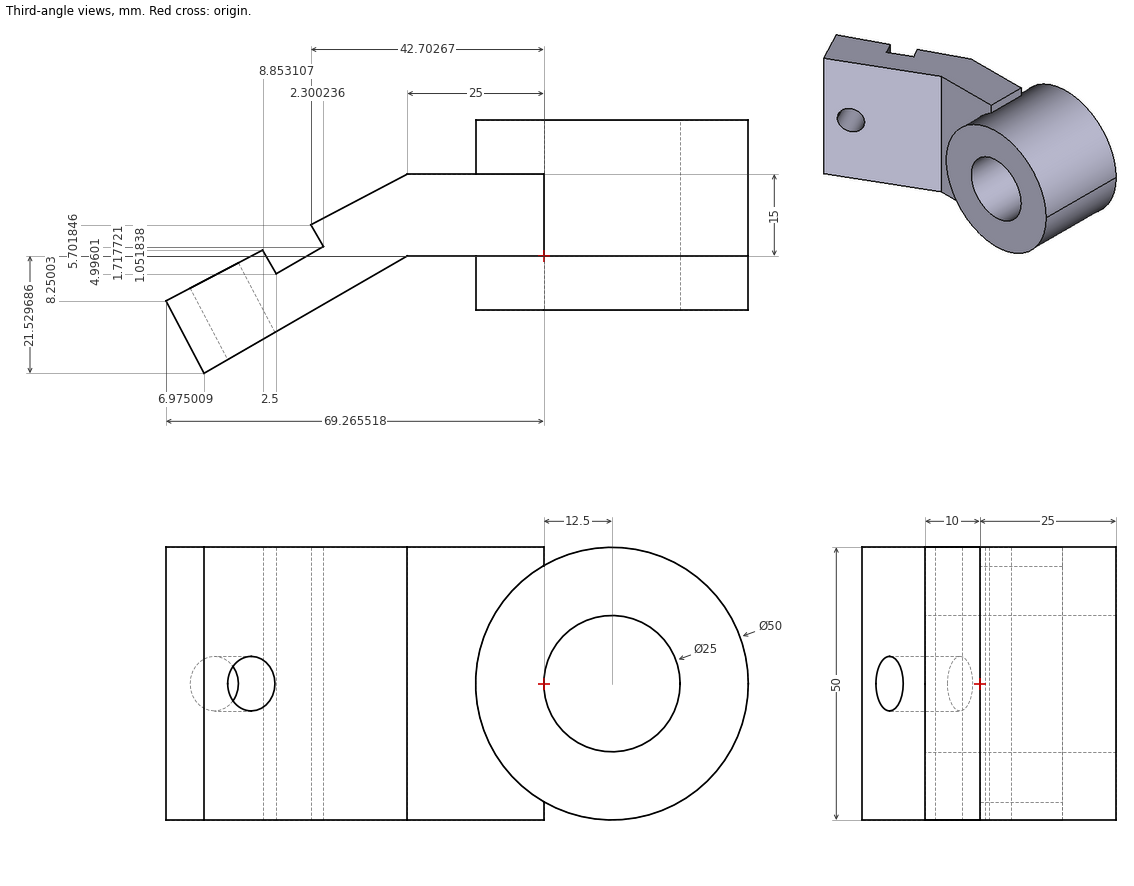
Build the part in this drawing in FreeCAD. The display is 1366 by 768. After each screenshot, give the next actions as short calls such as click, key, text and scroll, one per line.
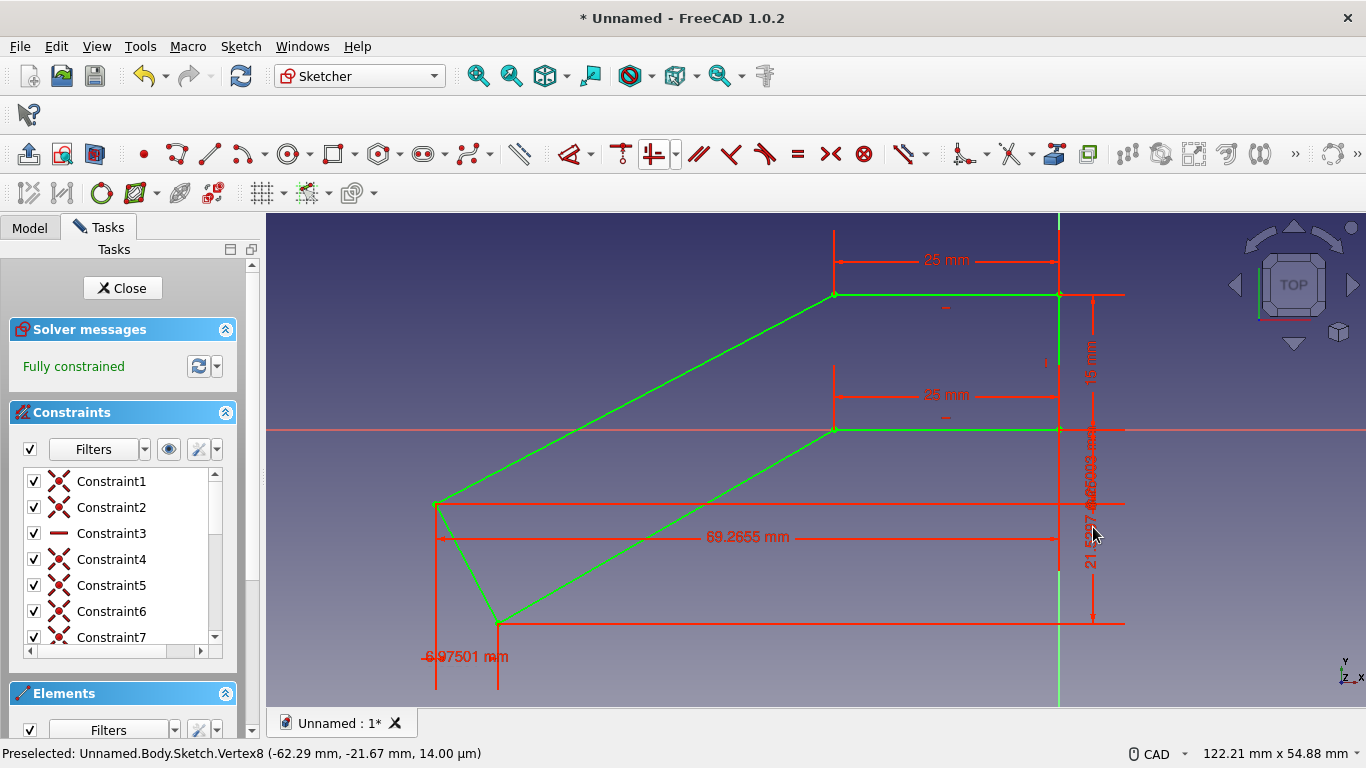
click(123, 288)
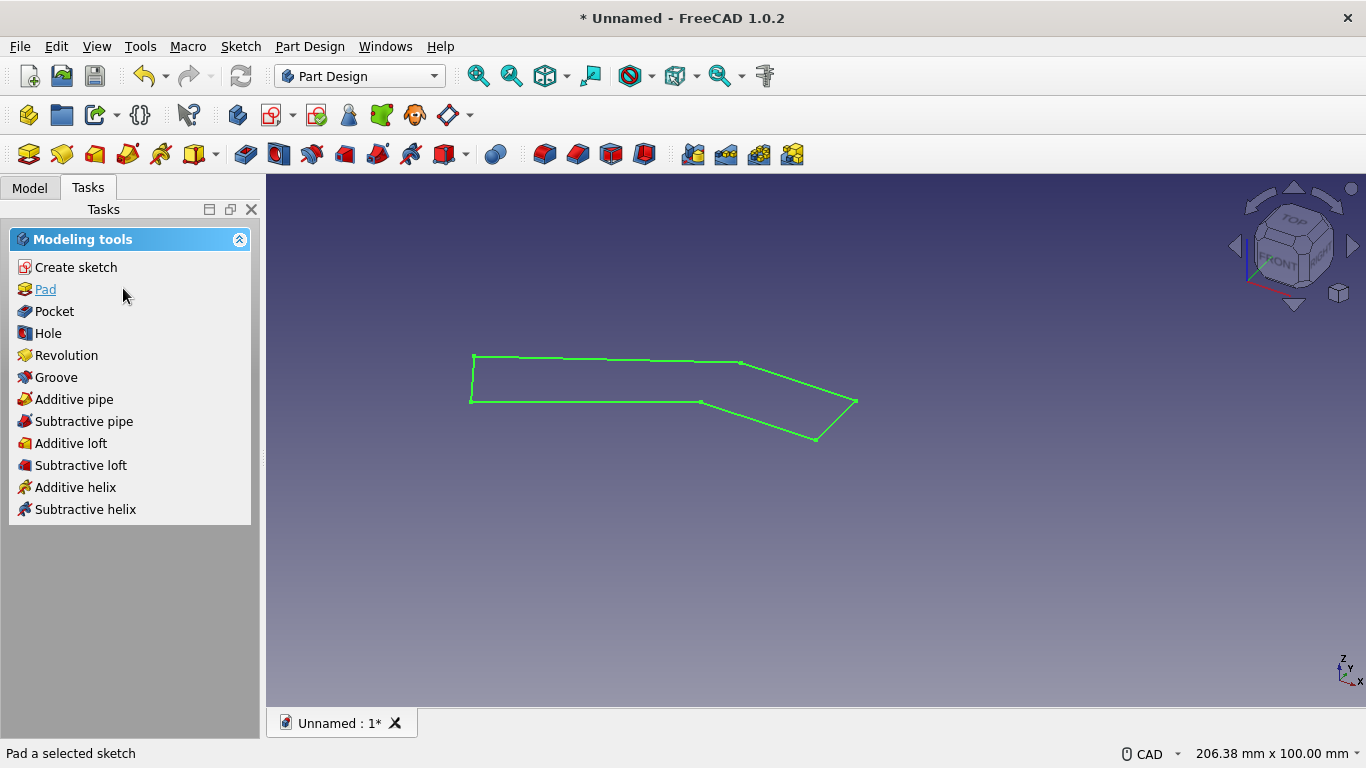
click(29, 154)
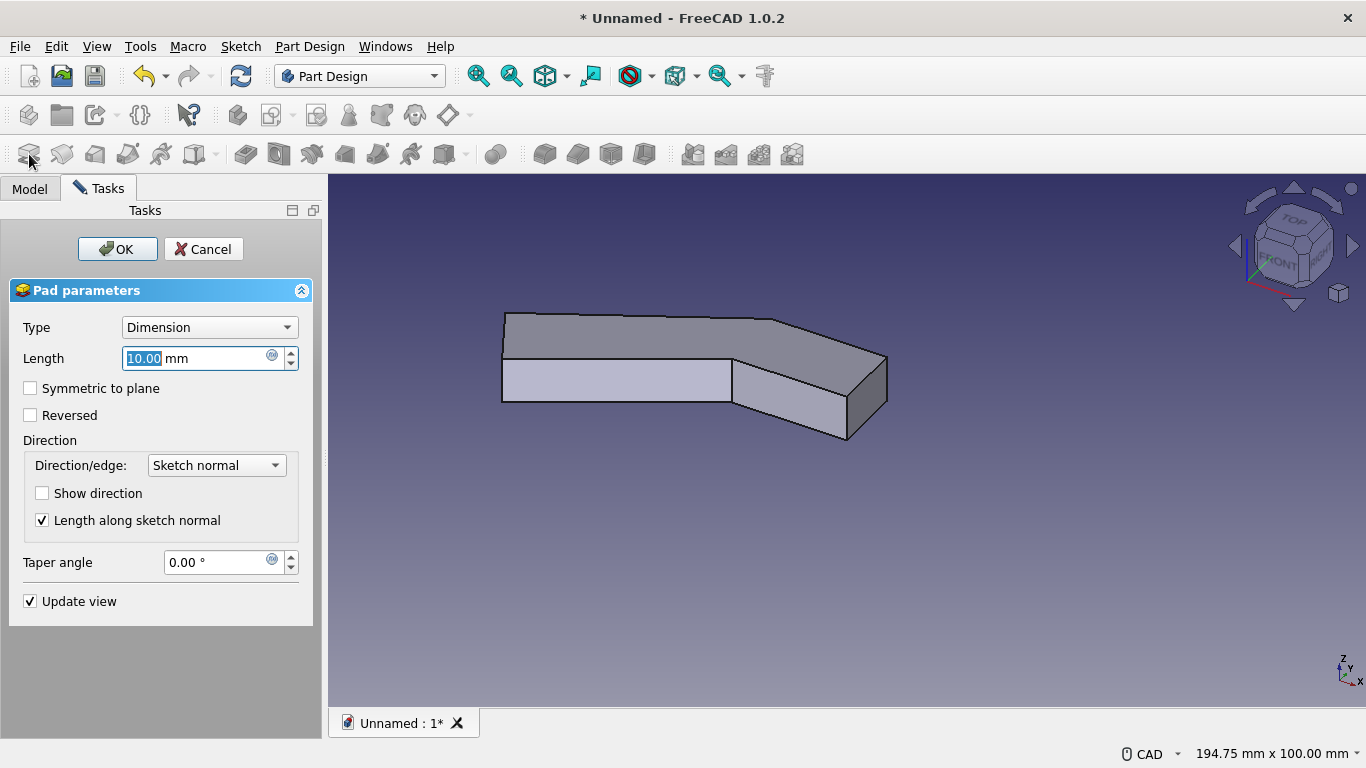
text(50)
key(Tab)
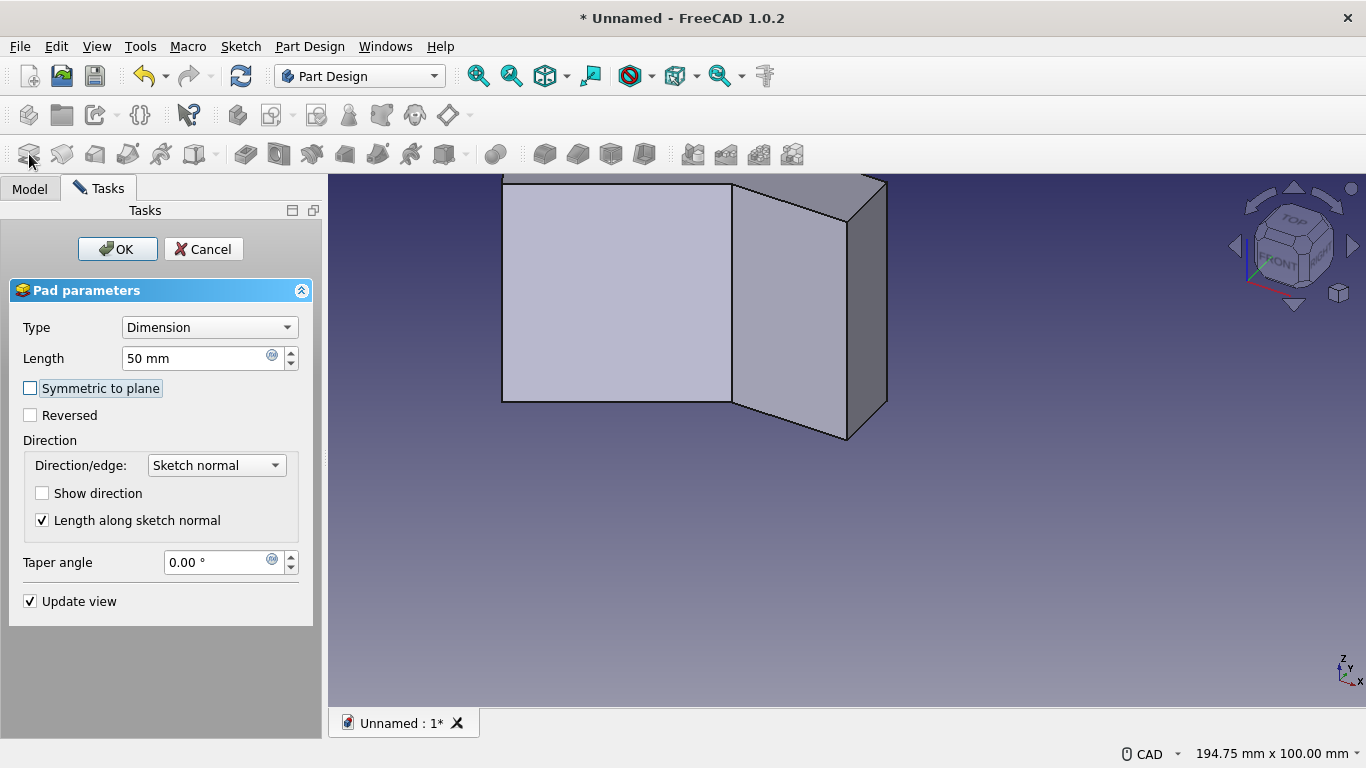
click(31, 388)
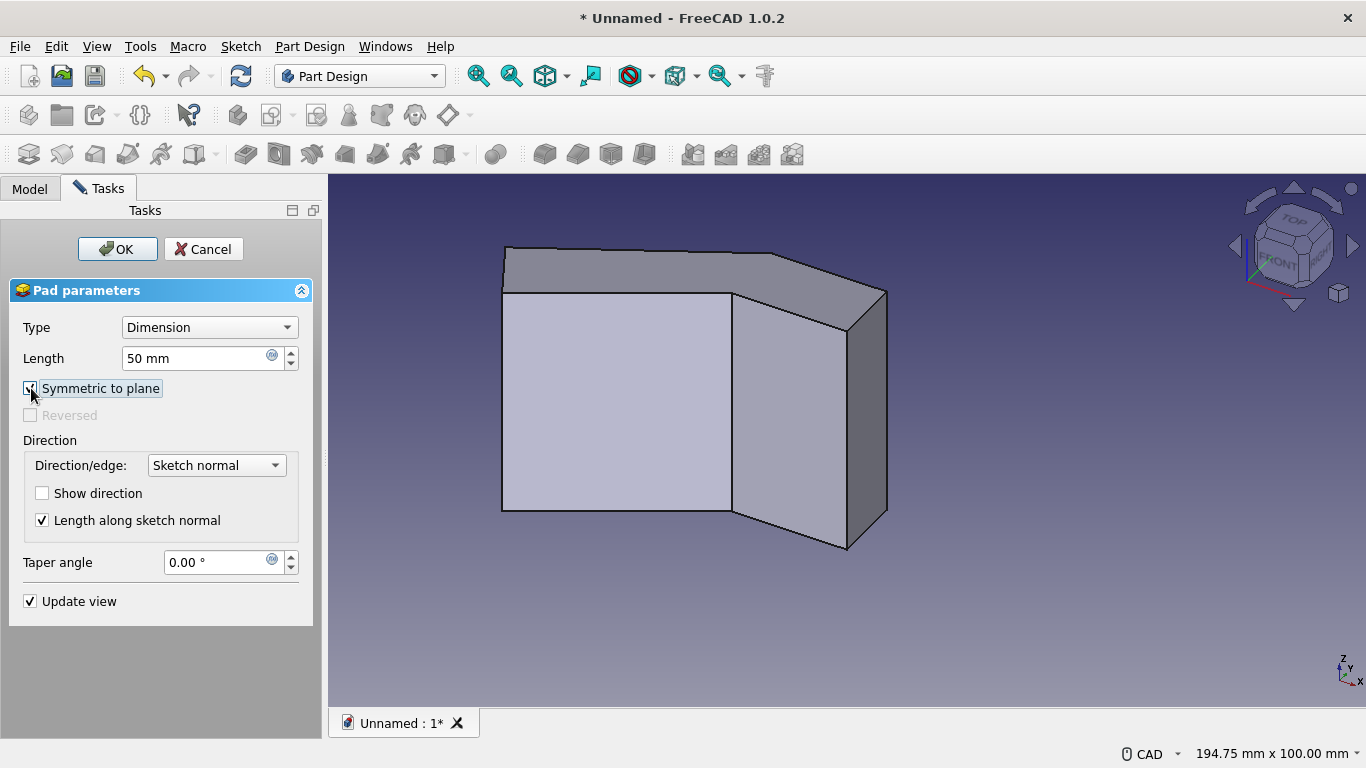
click(118, 249)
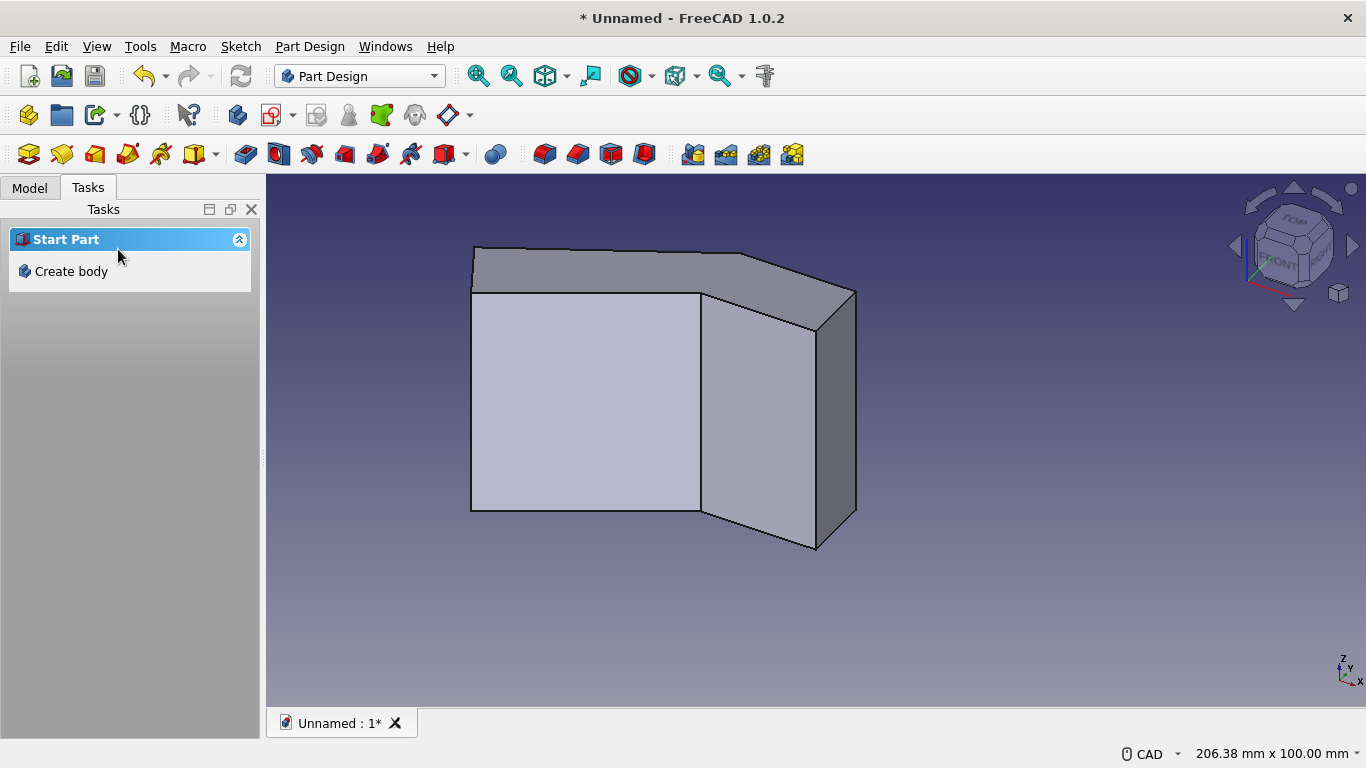
click(270, 116)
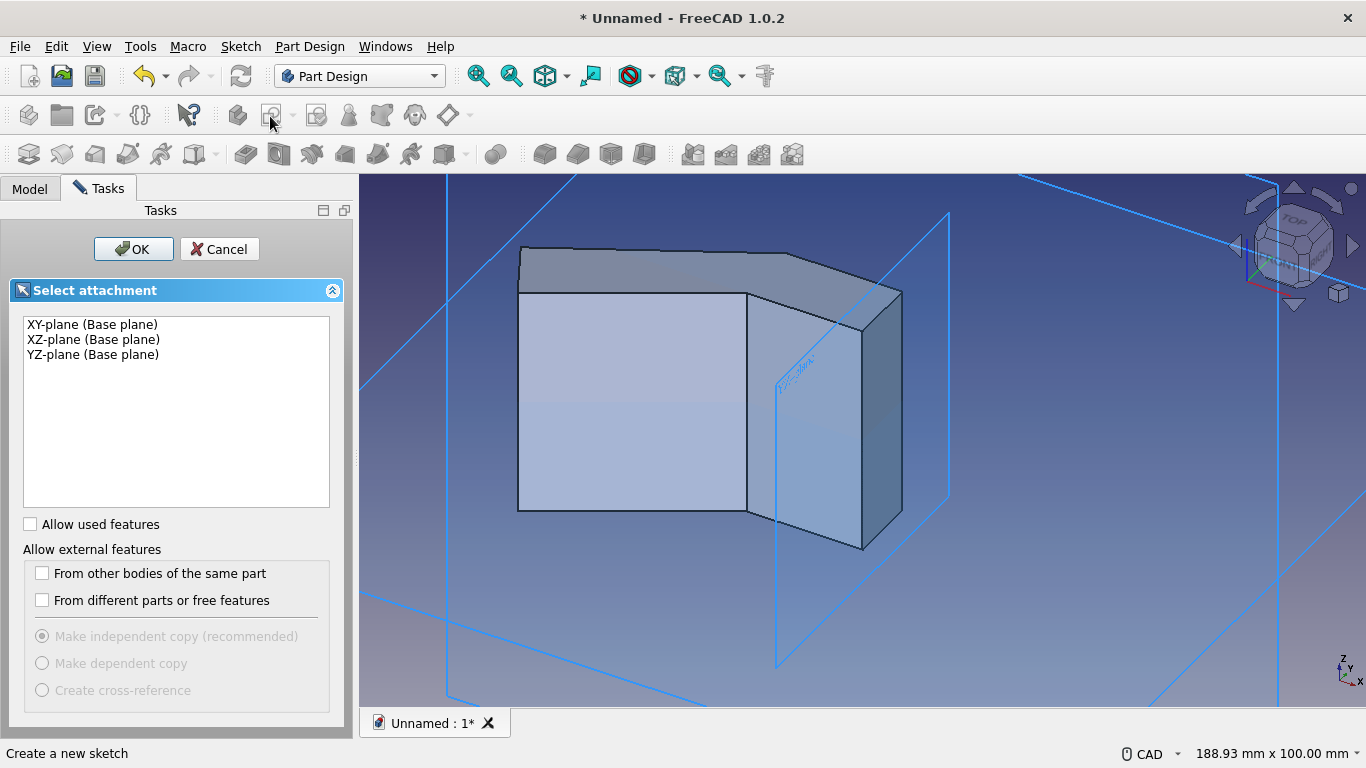
click(84, 340)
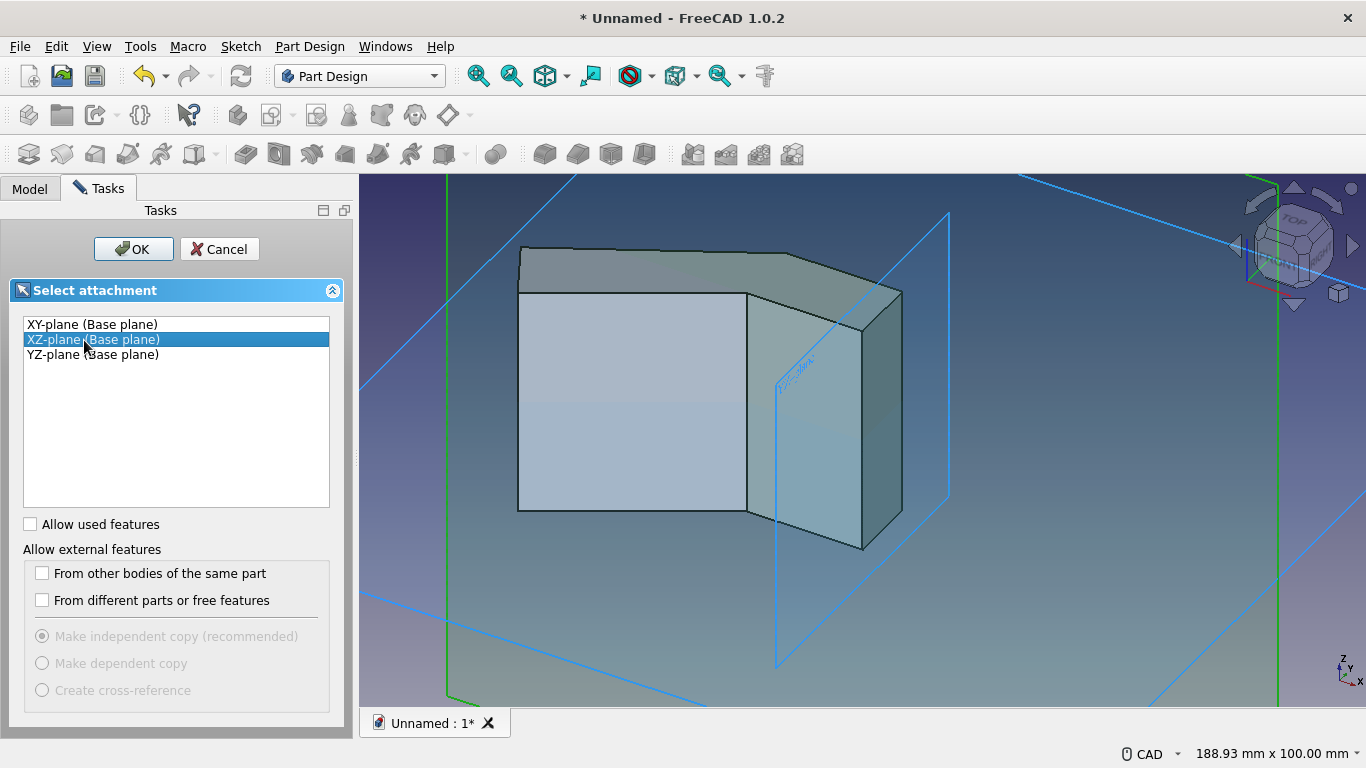
click(134, 249)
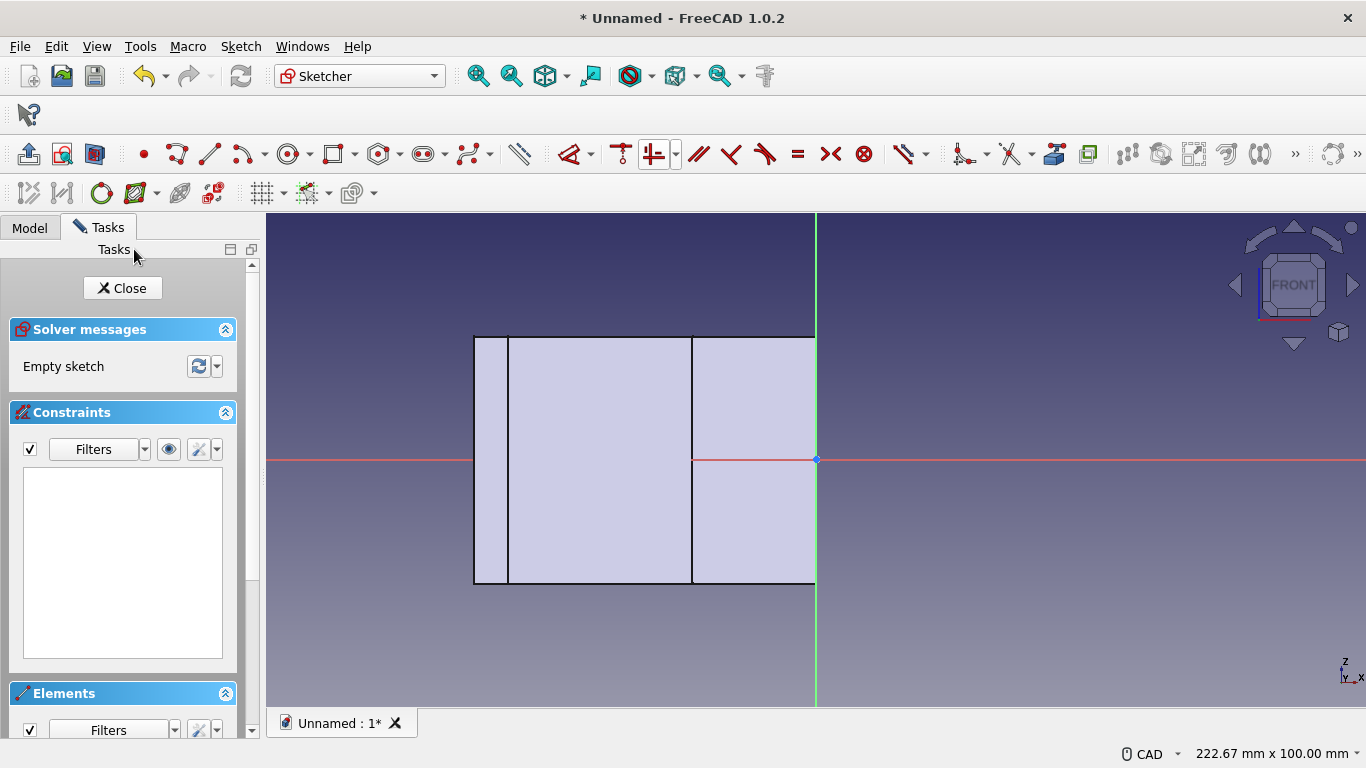
key(q)
key(s)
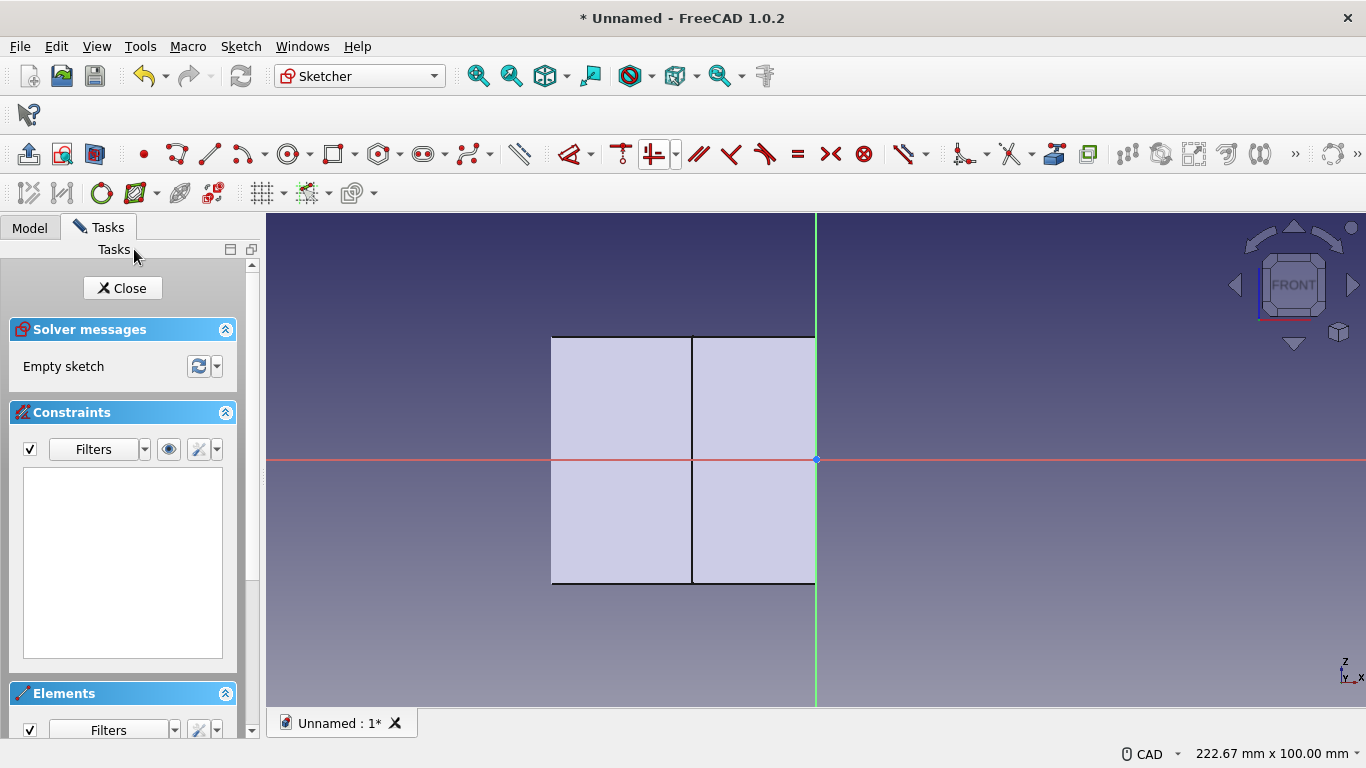
click(288, 154)